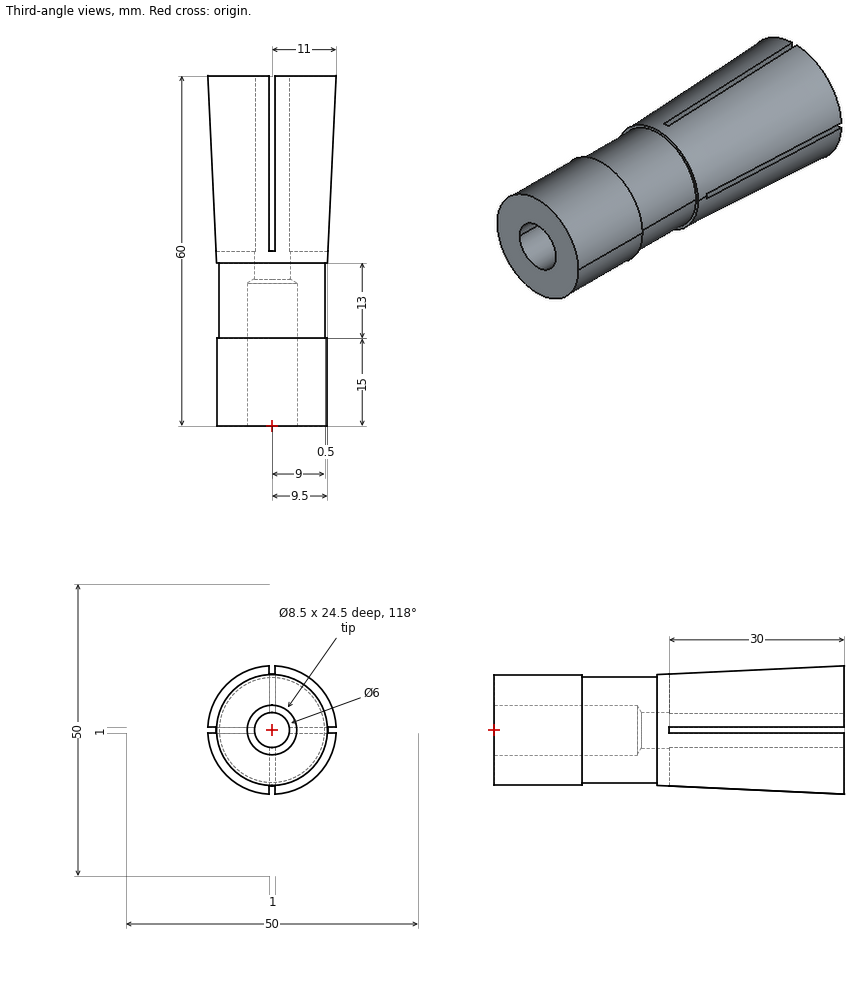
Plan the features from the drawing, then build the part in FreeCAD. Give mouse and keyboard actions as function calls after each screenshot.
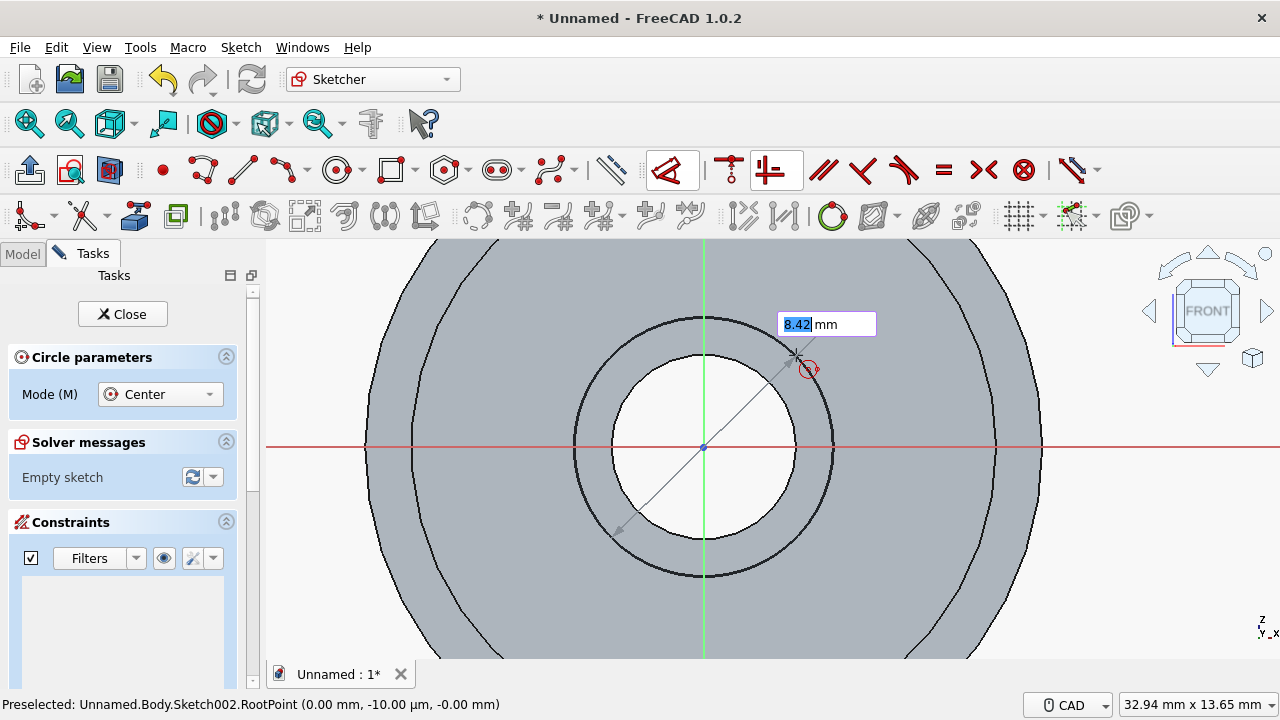
text(8.5)
key(Return)
key(Escape)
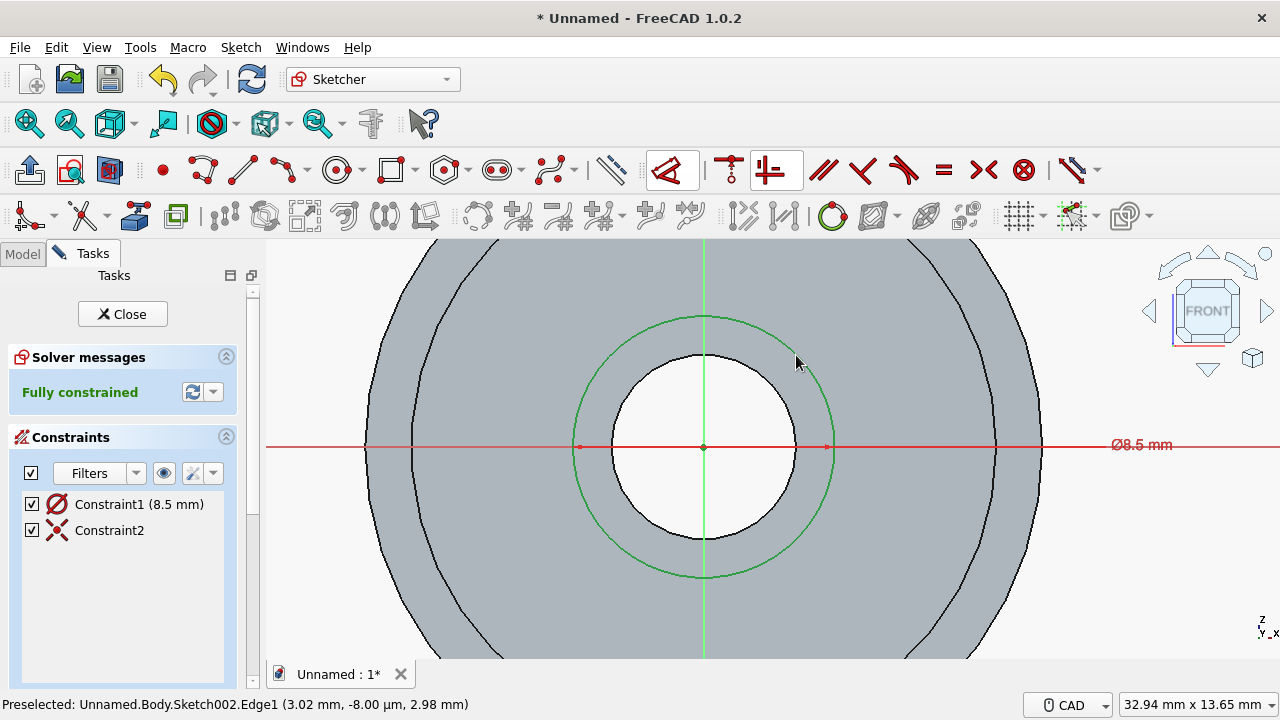
click(123, 314)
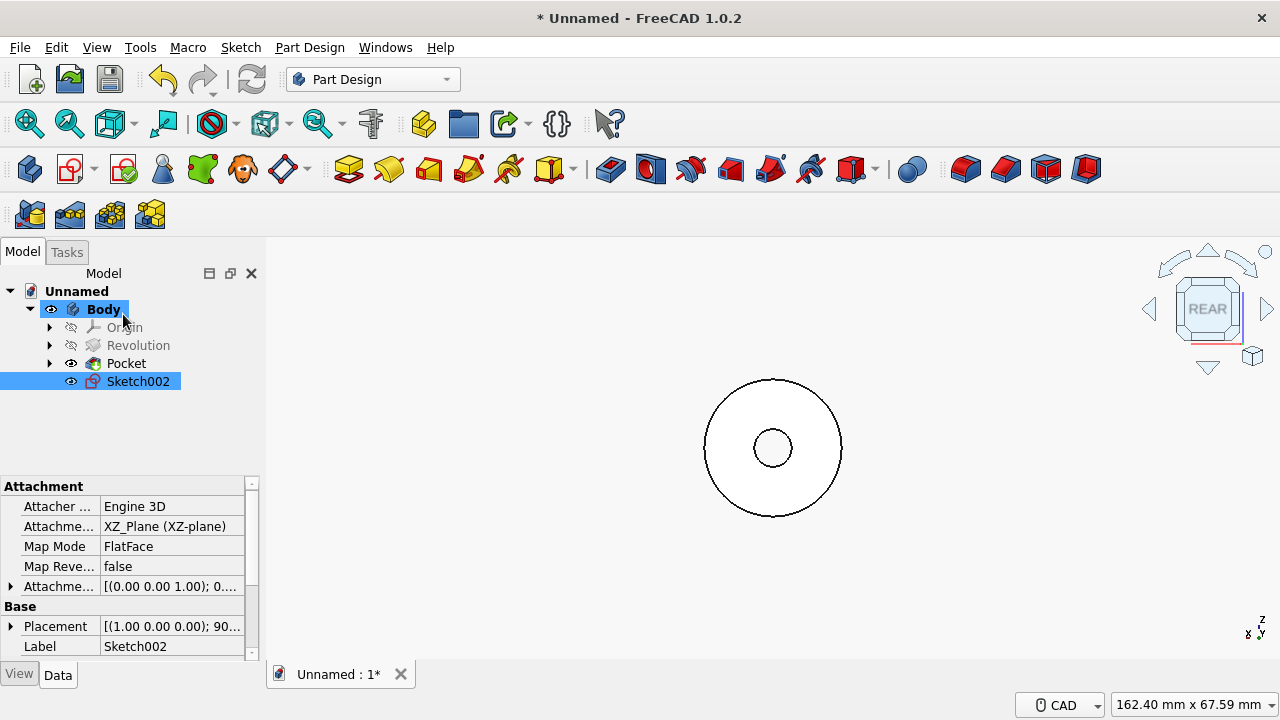
click(652, 170)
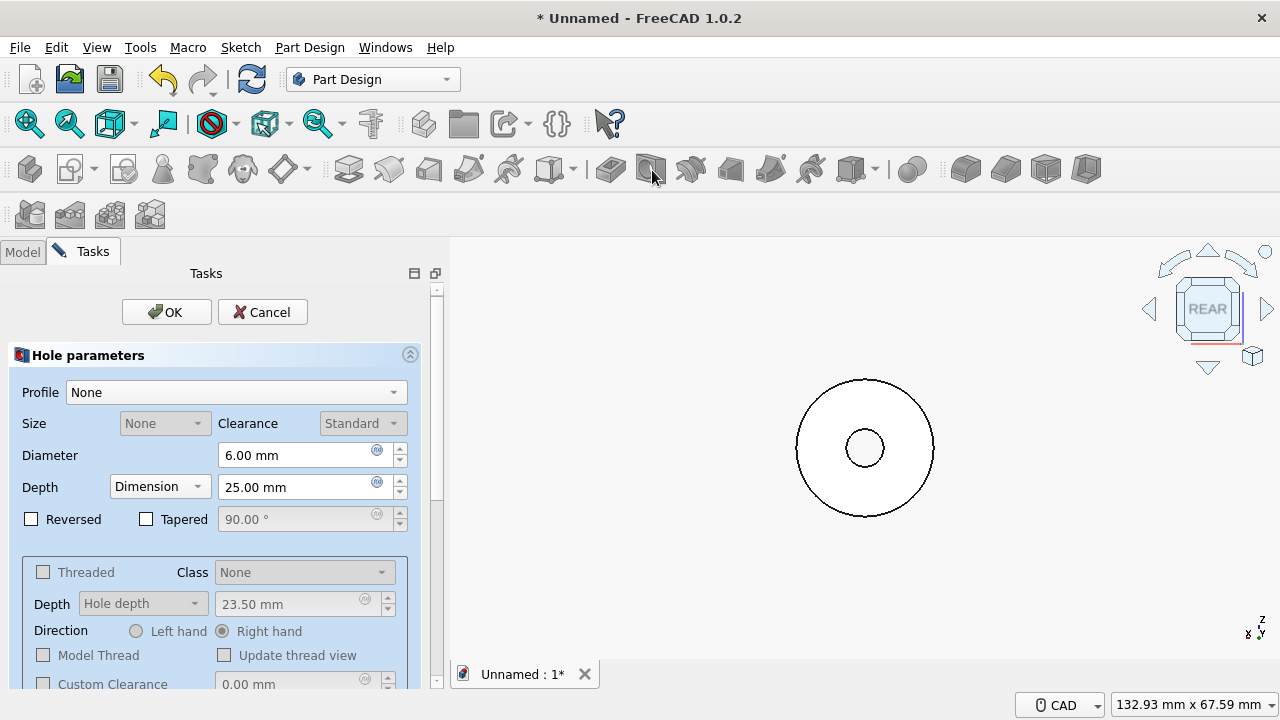
triple_click(305, 455)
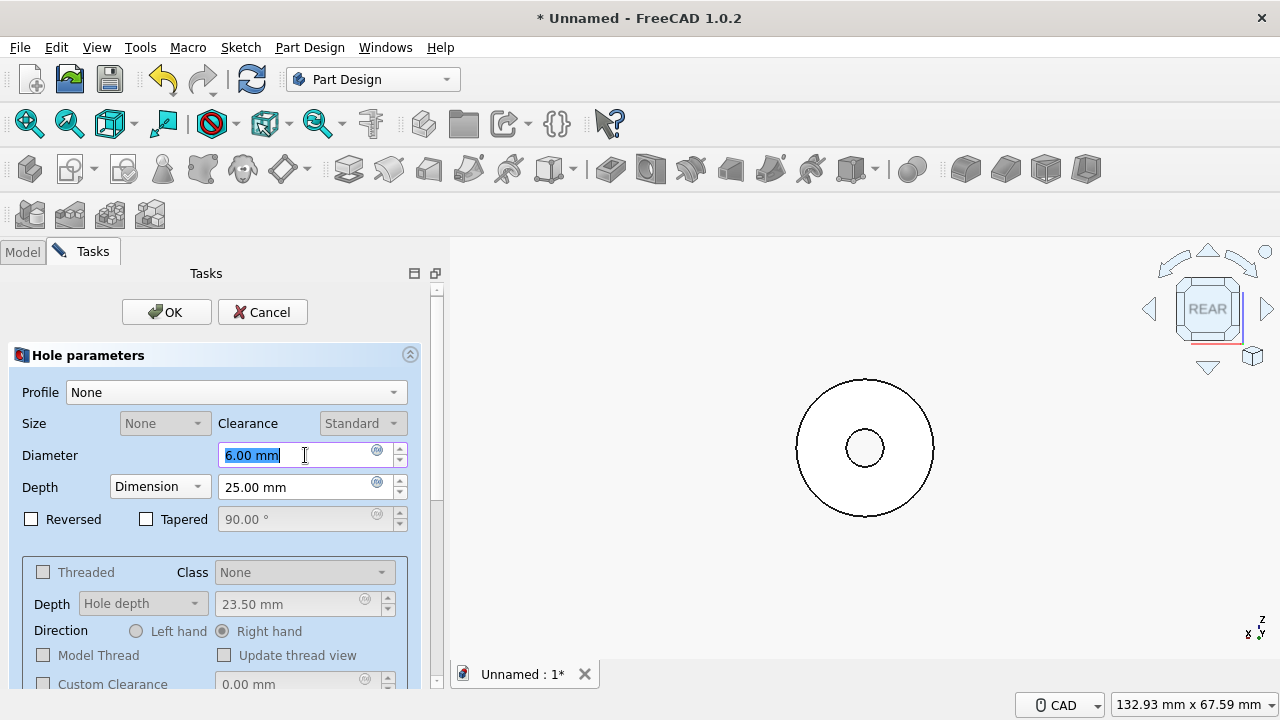
text(8.5)
key(Tab)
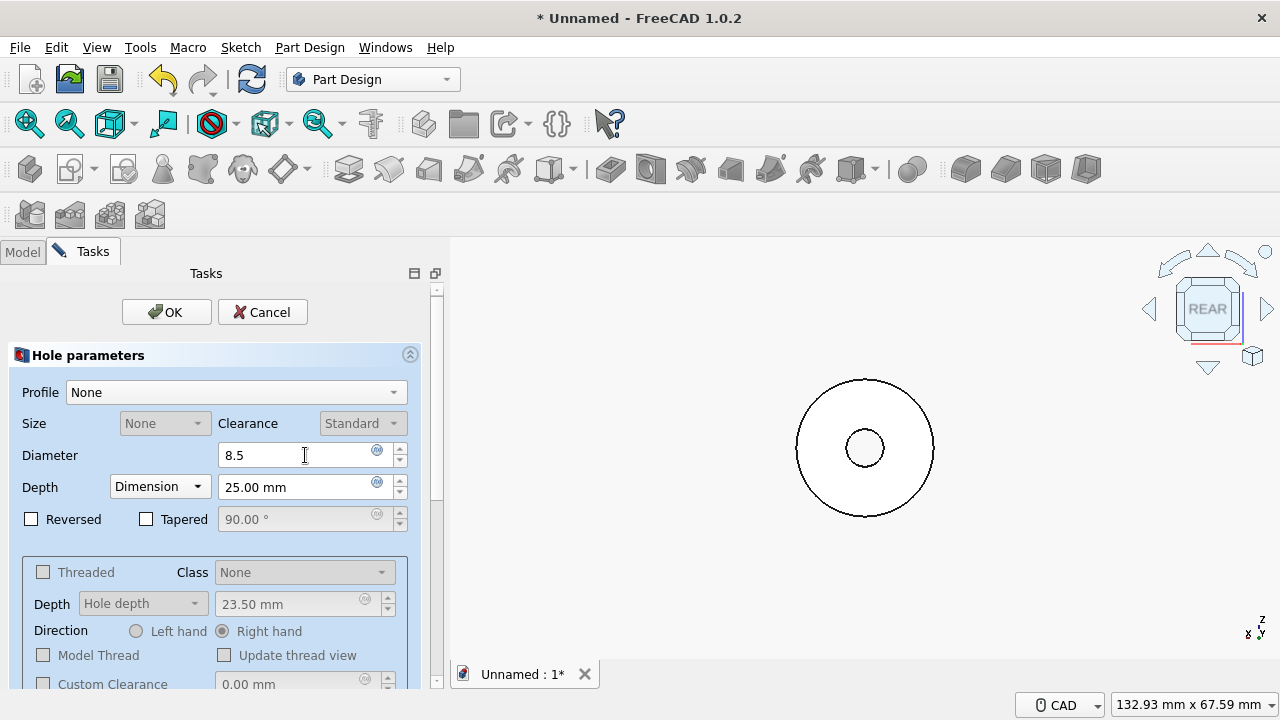
triple_click(305, 487)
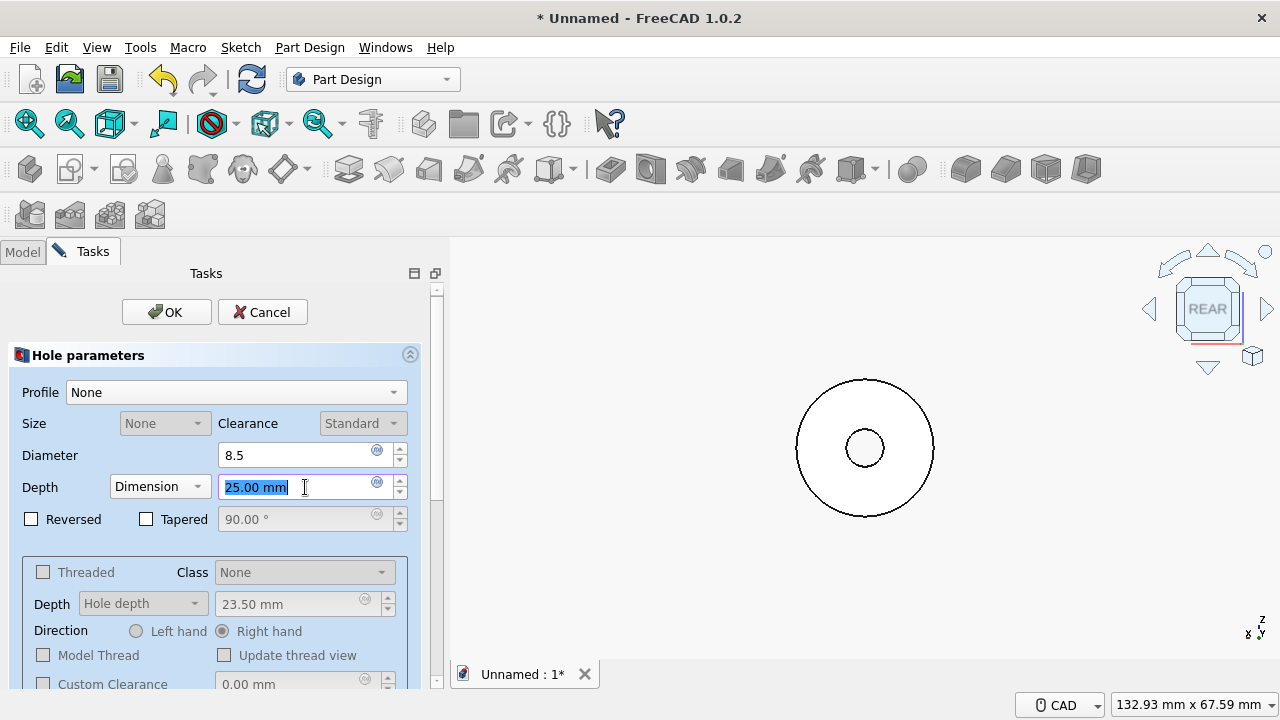
text(24.5)
key(Tab)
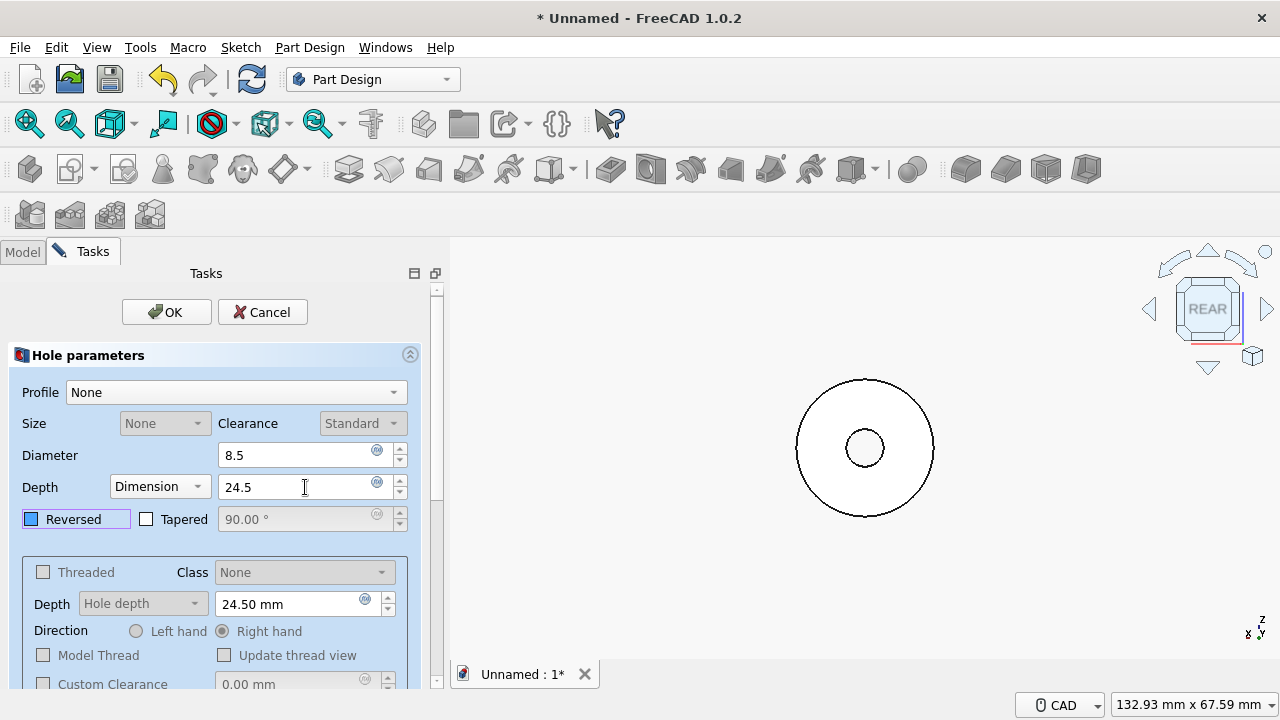
click(167, 312)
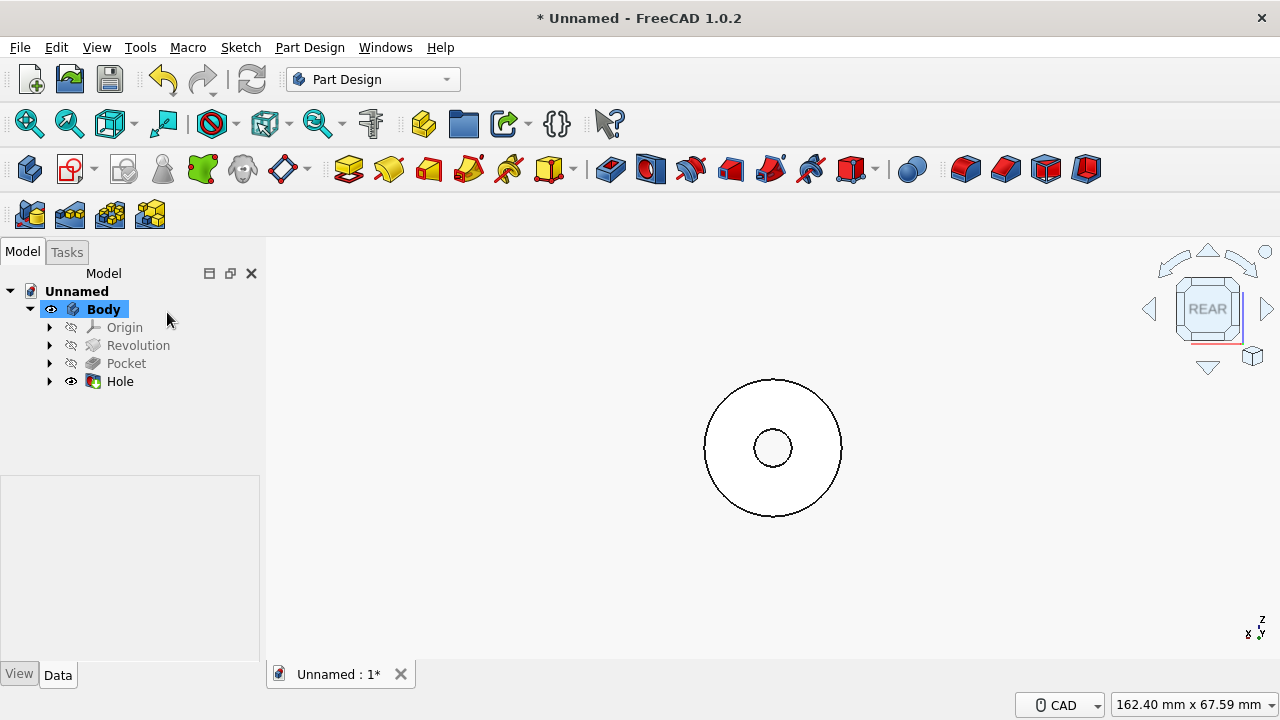
click(30, 124)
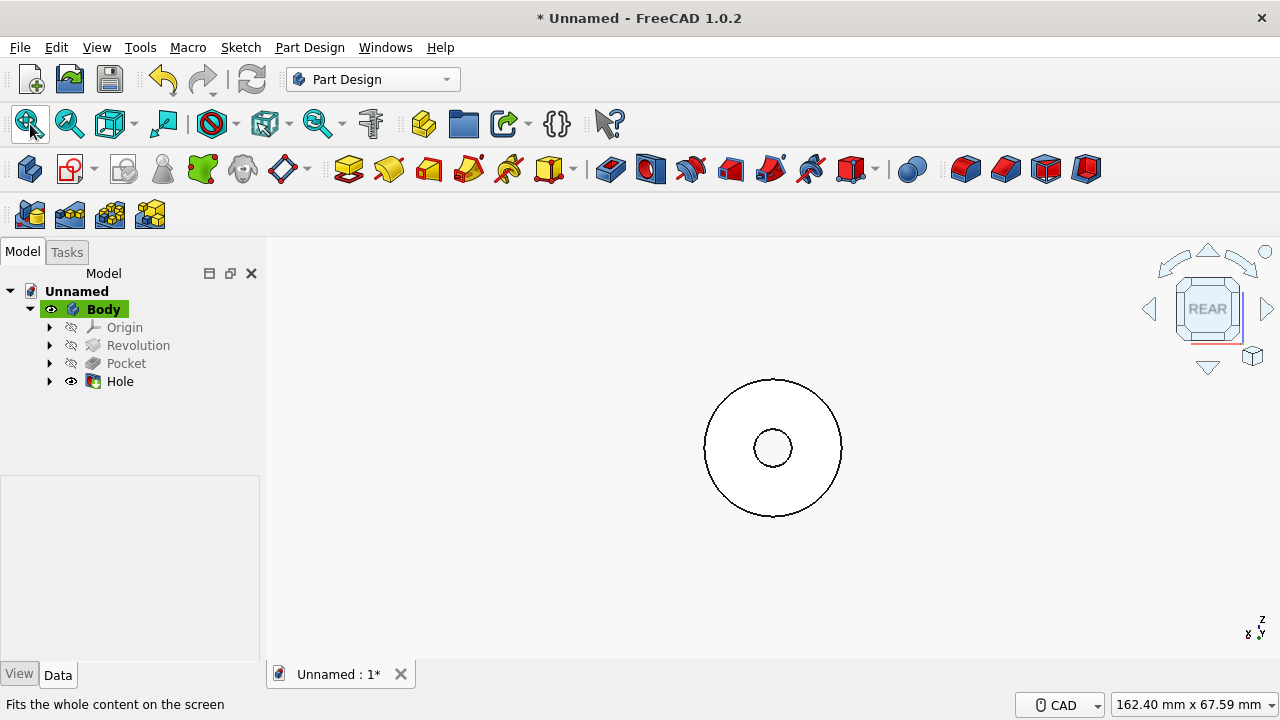
click(753, 408)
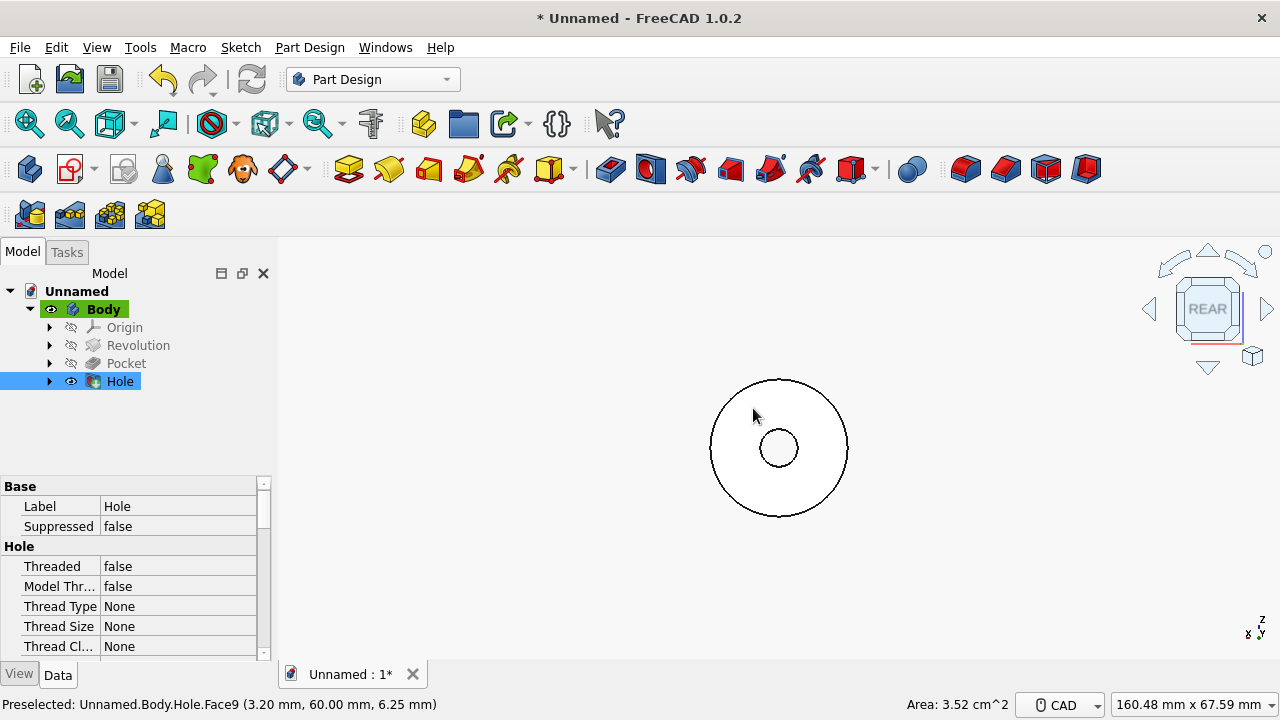
click(70, 170)